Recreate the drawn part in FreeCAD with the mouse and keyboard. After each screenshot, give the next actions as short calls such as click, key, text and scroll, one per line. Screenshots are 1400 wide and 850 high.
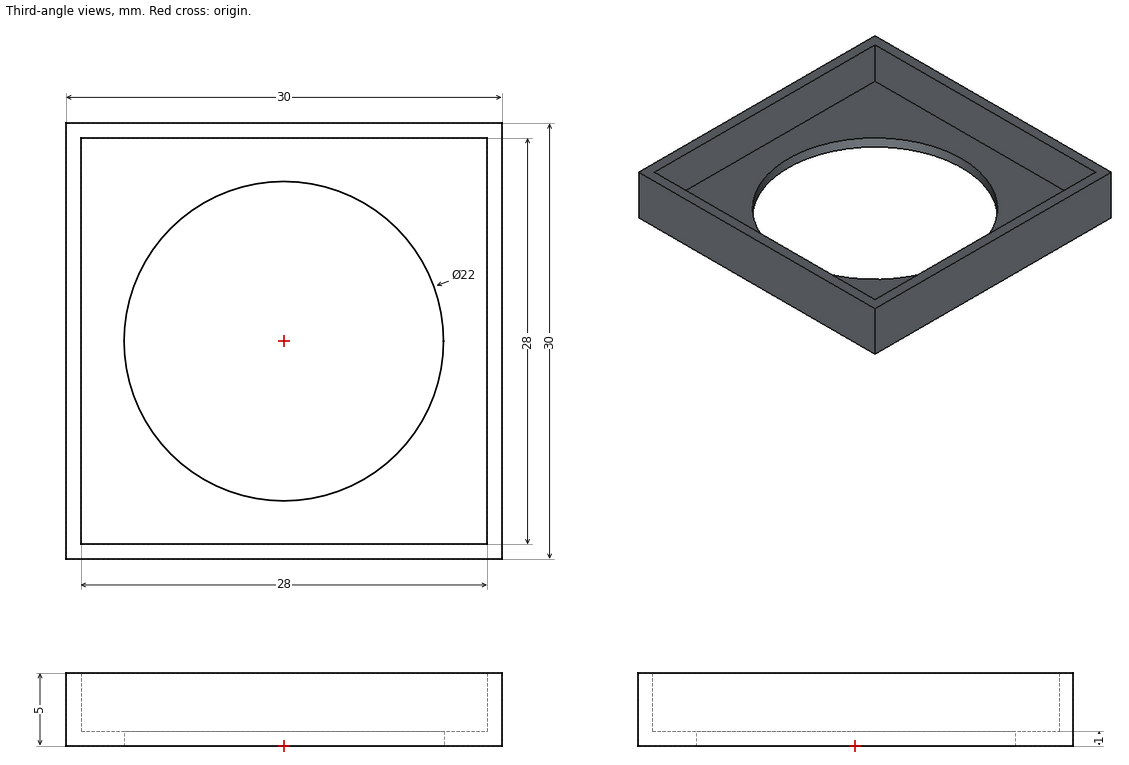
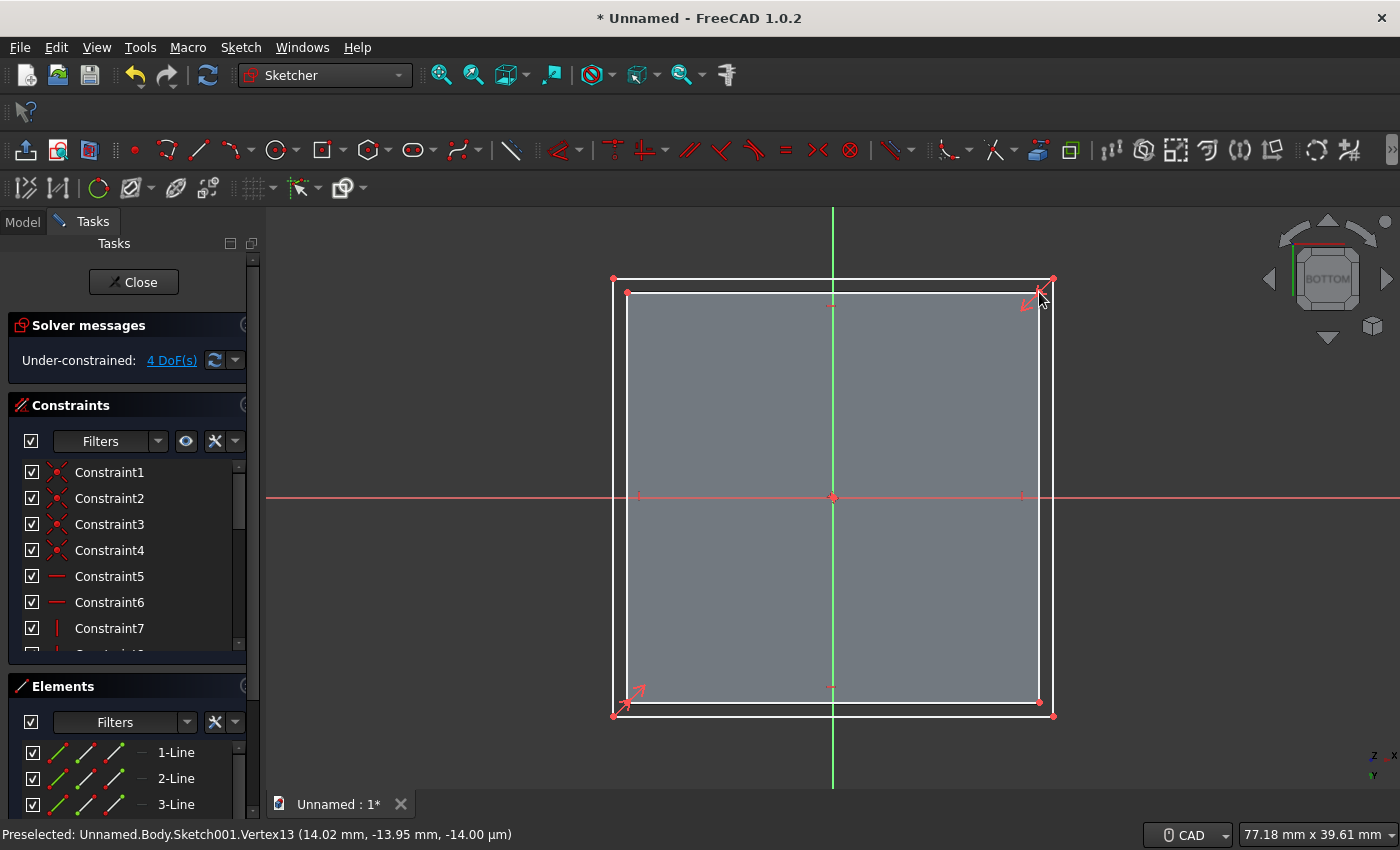
click(558, 150)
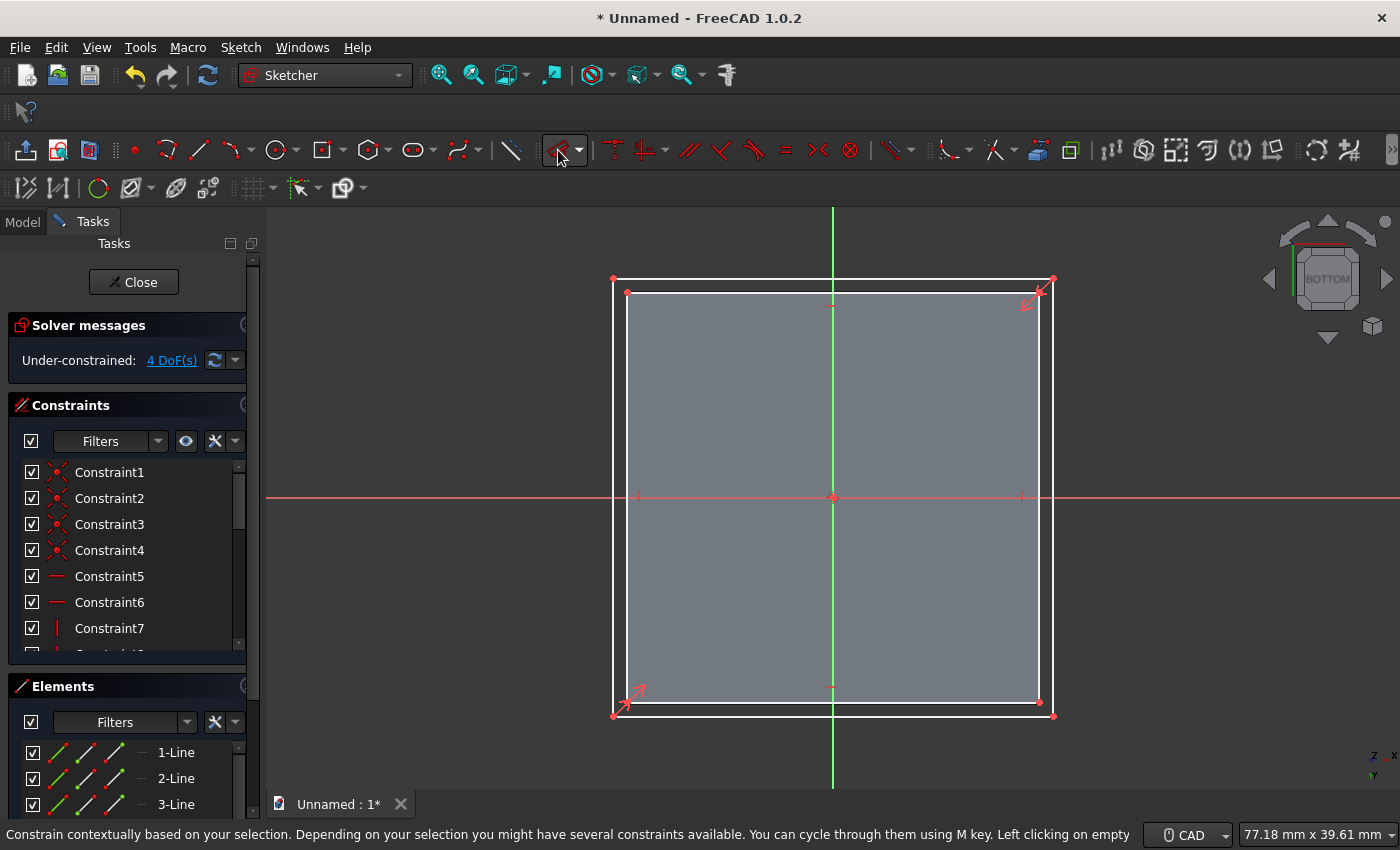
click(745, 717)
click(732, 751)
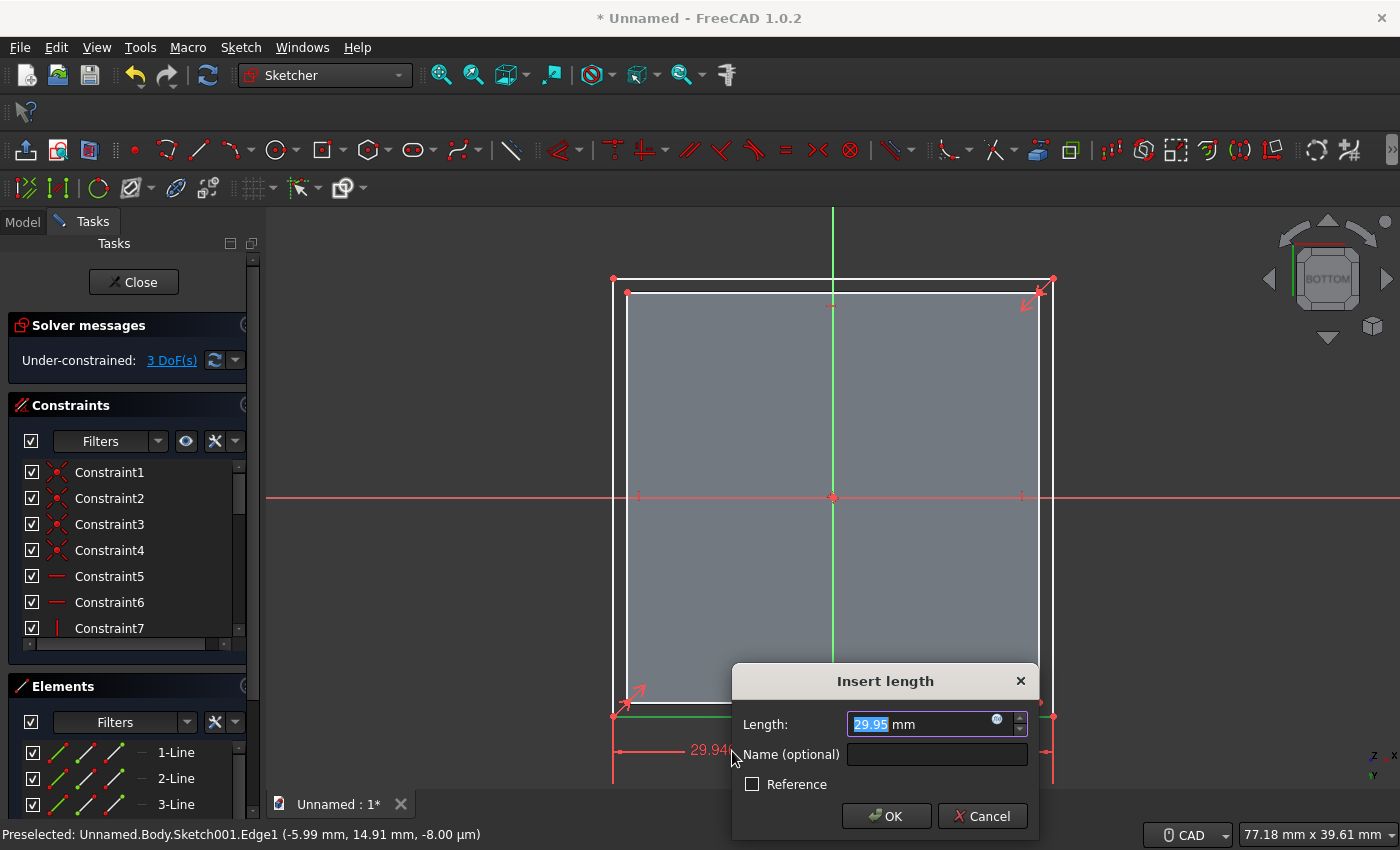
text(30)
key(Return)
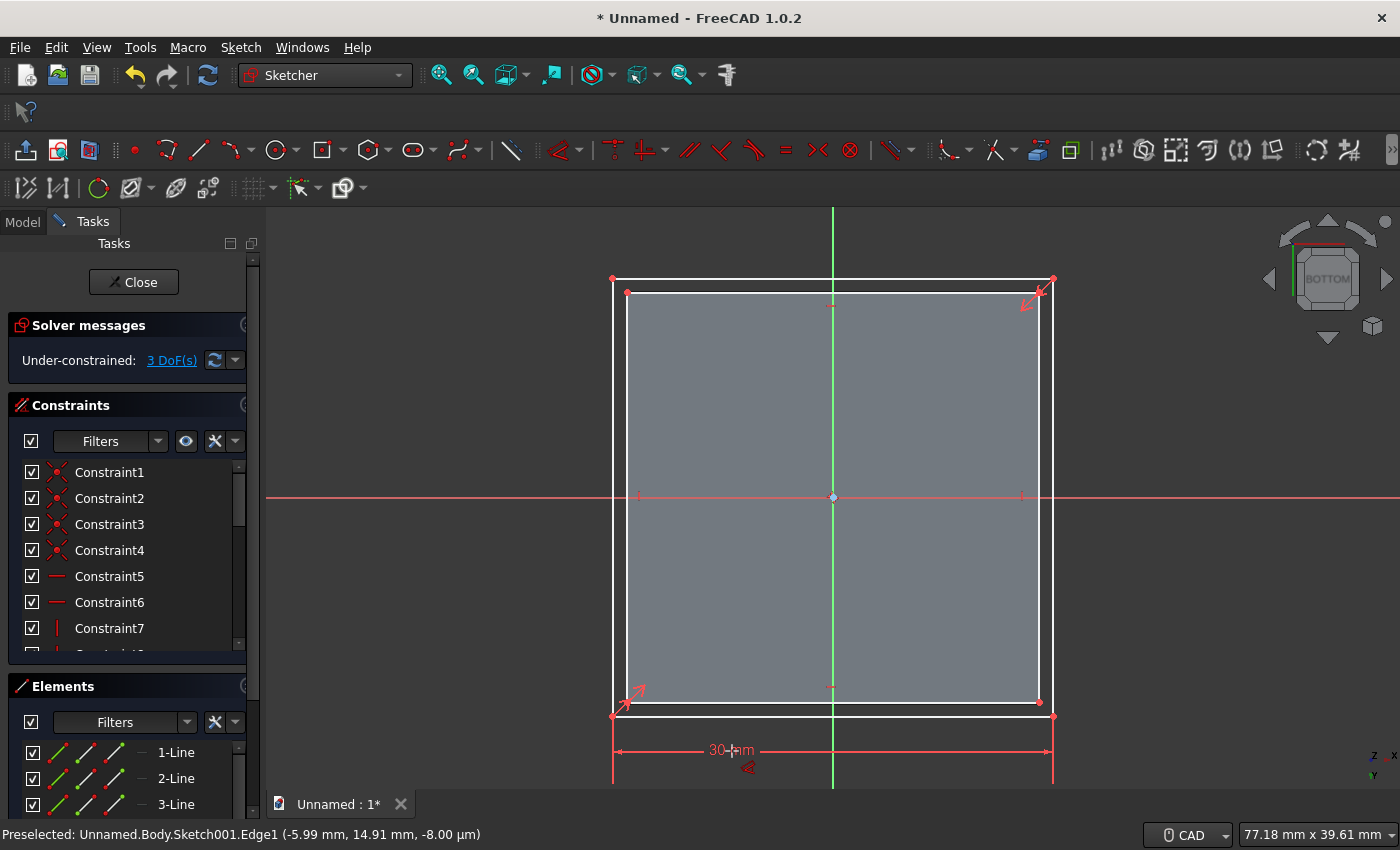
click(1053, 586)
click(1087, 397)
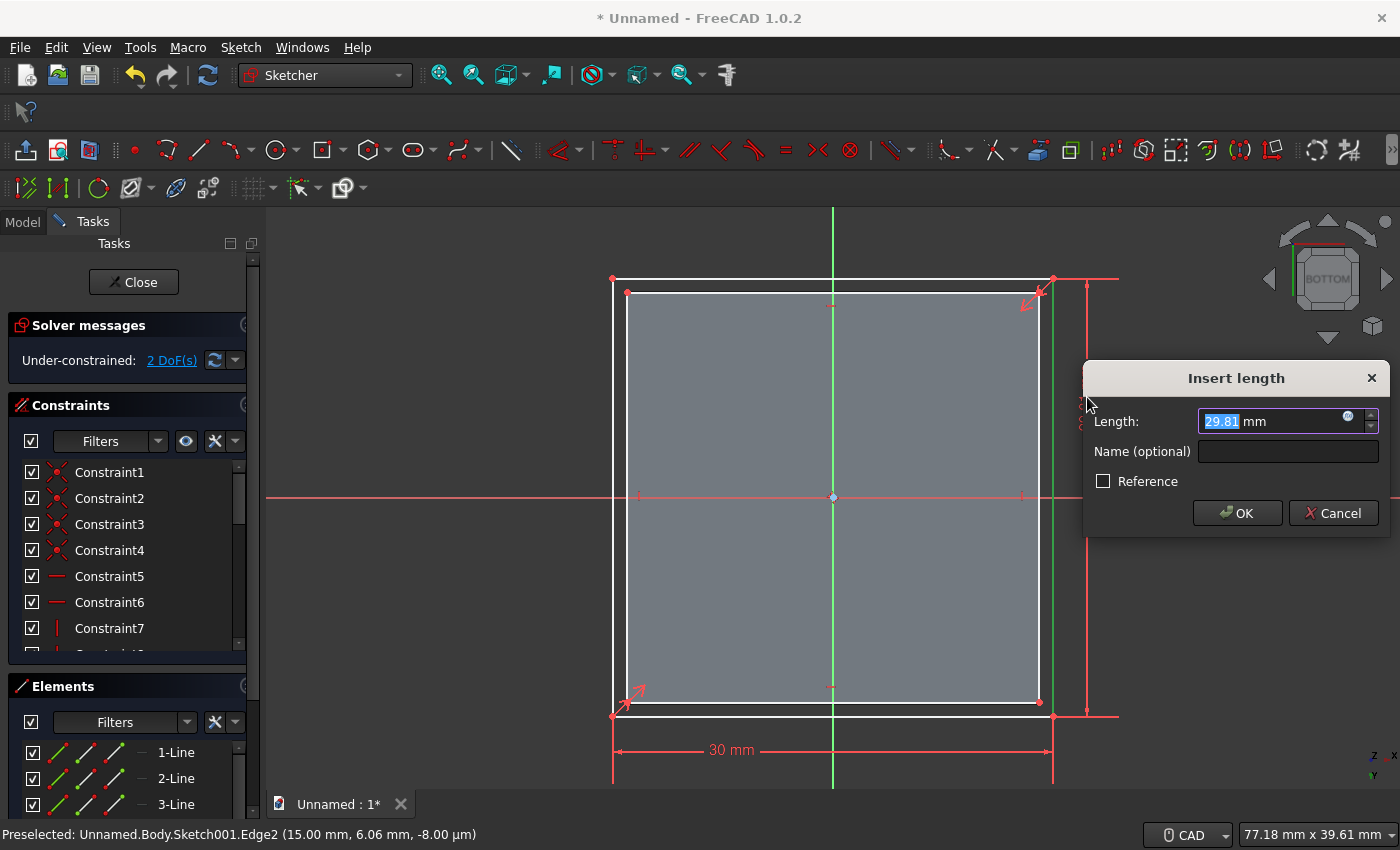
text(30)
key(Return)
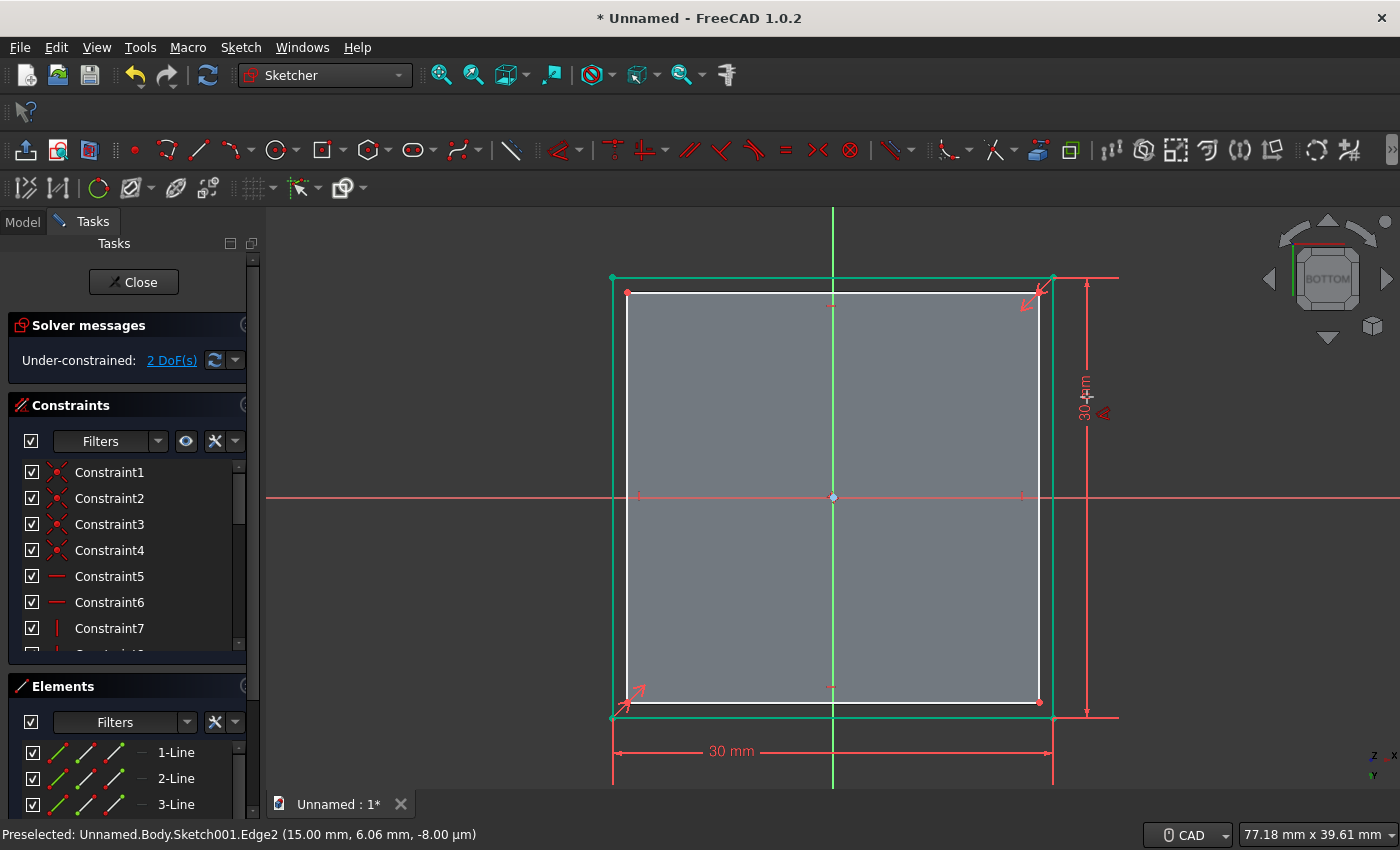
click(751, 703)
click(928, 737)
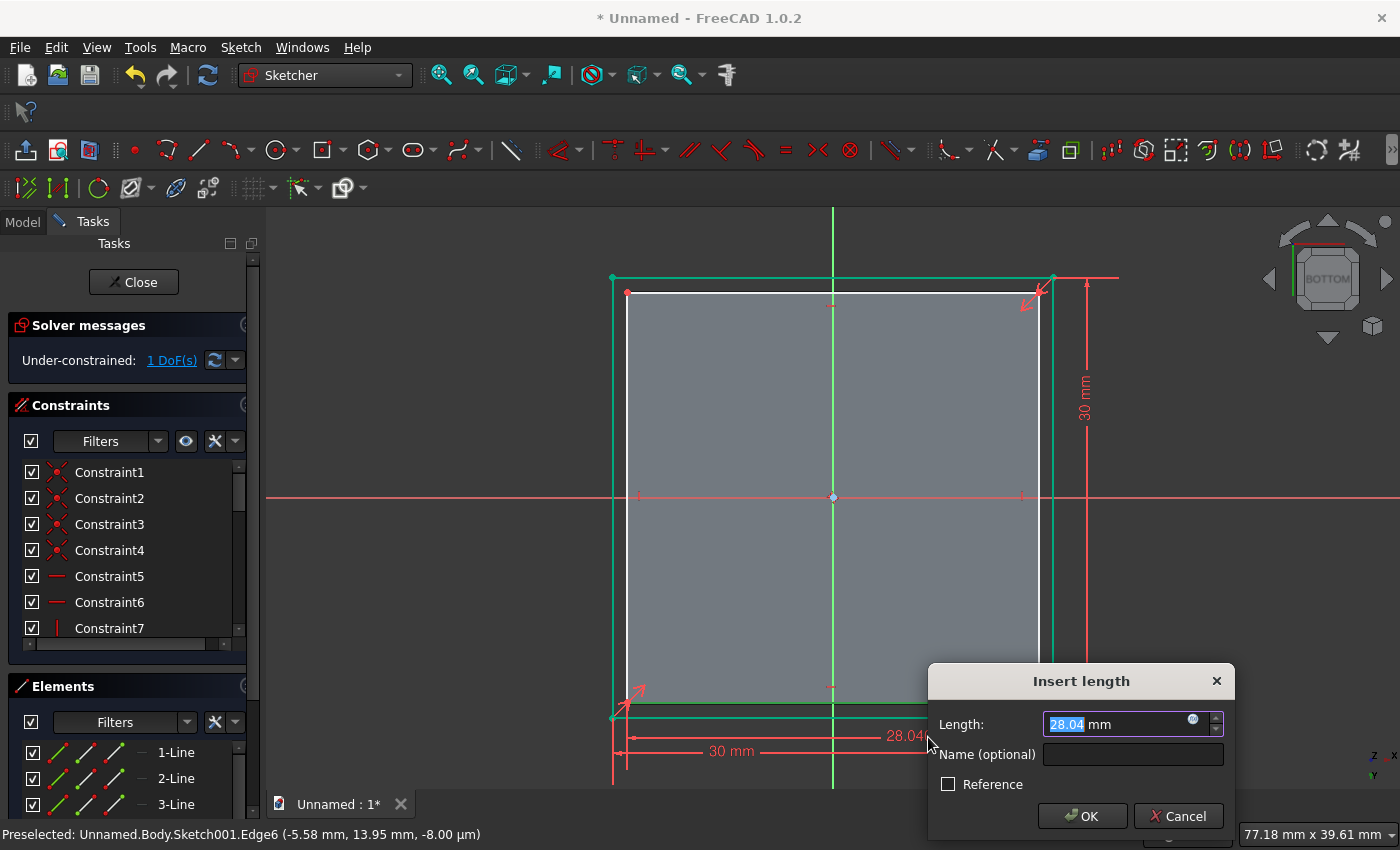
text(28)
key(Return)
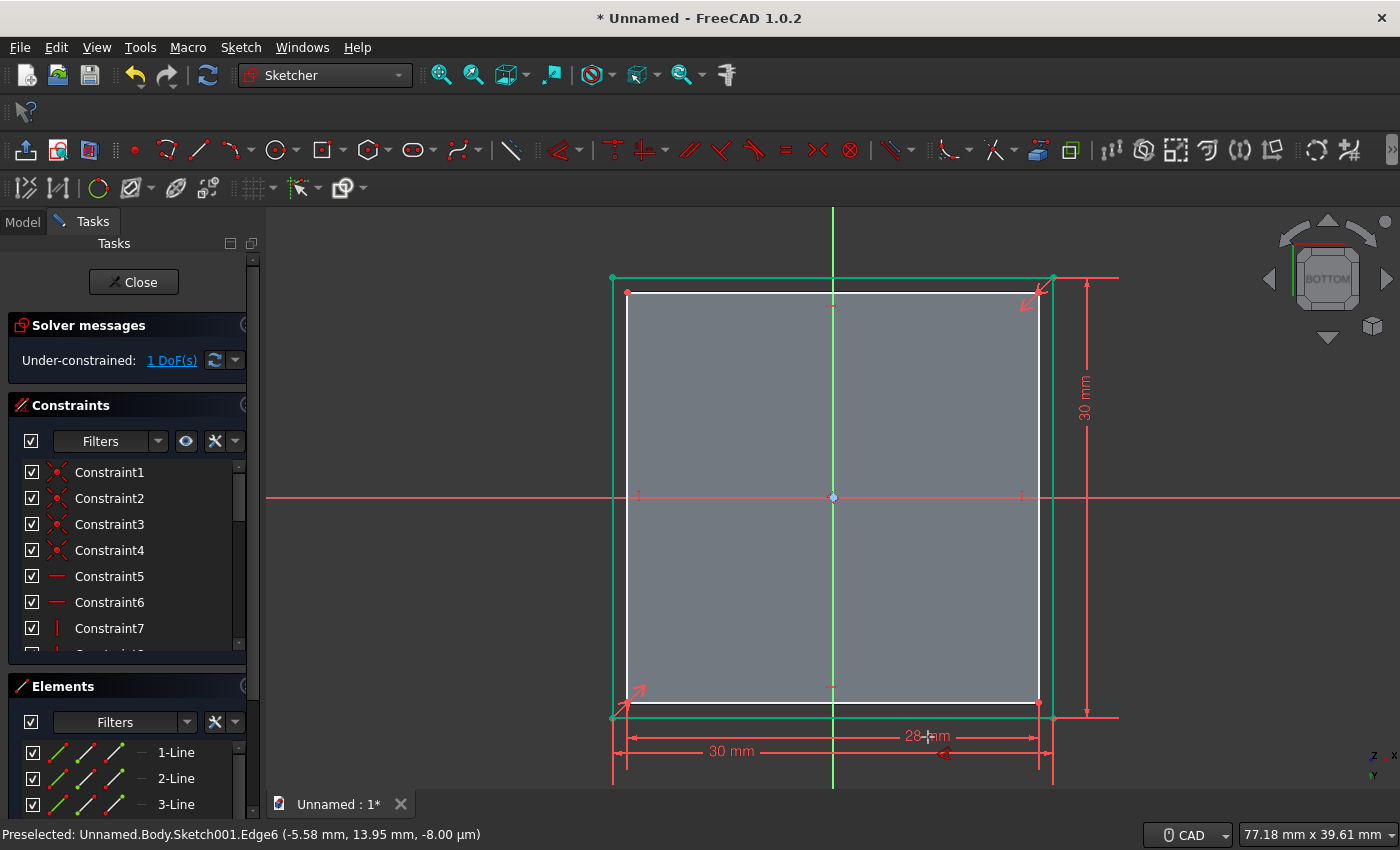
click(1039, 580)
click(1073, 592)